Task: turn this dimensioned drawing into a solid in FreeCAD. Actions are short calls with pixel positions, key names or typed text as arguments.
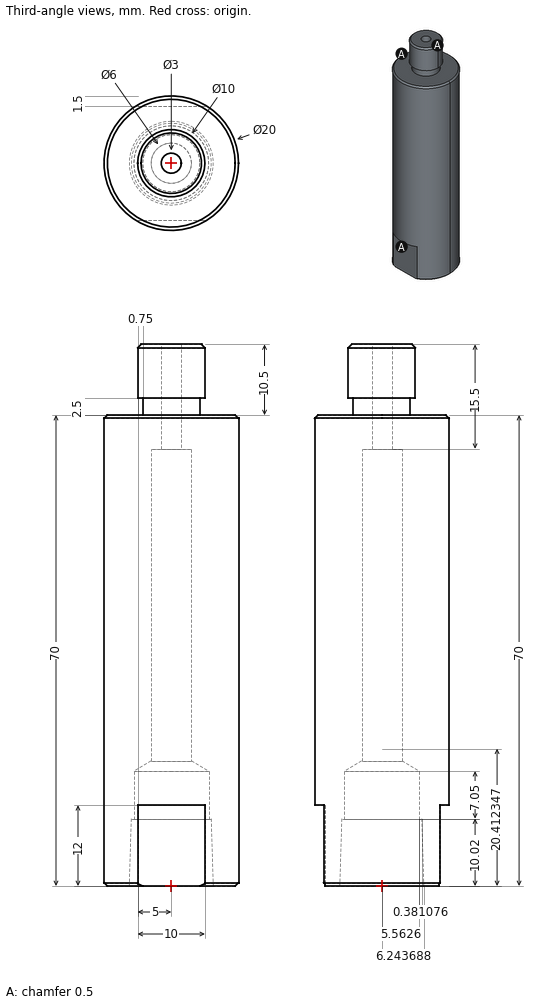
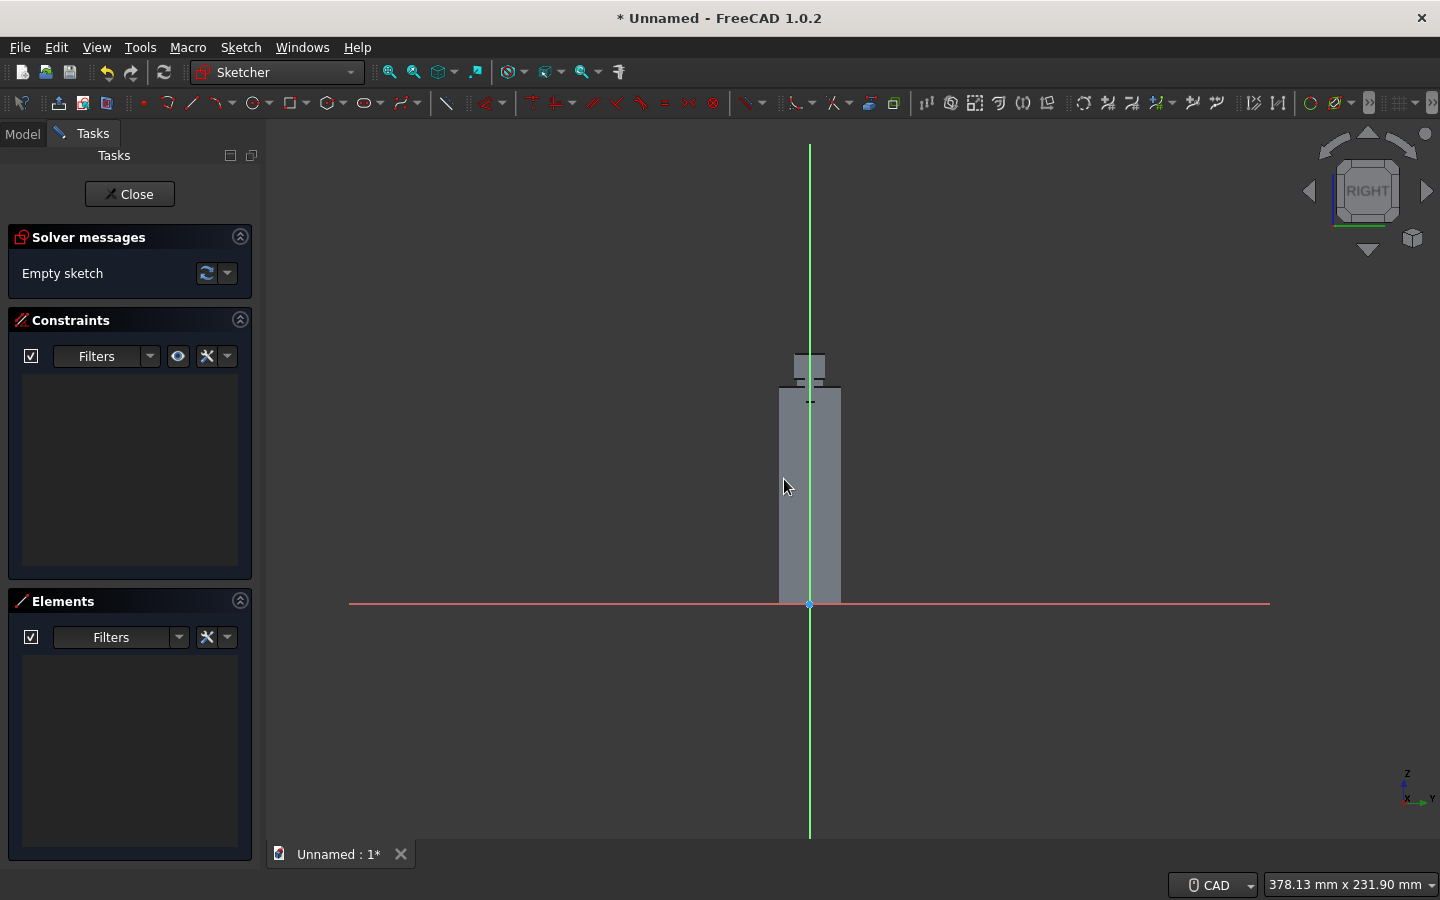
scroll(825, 587, up, 10)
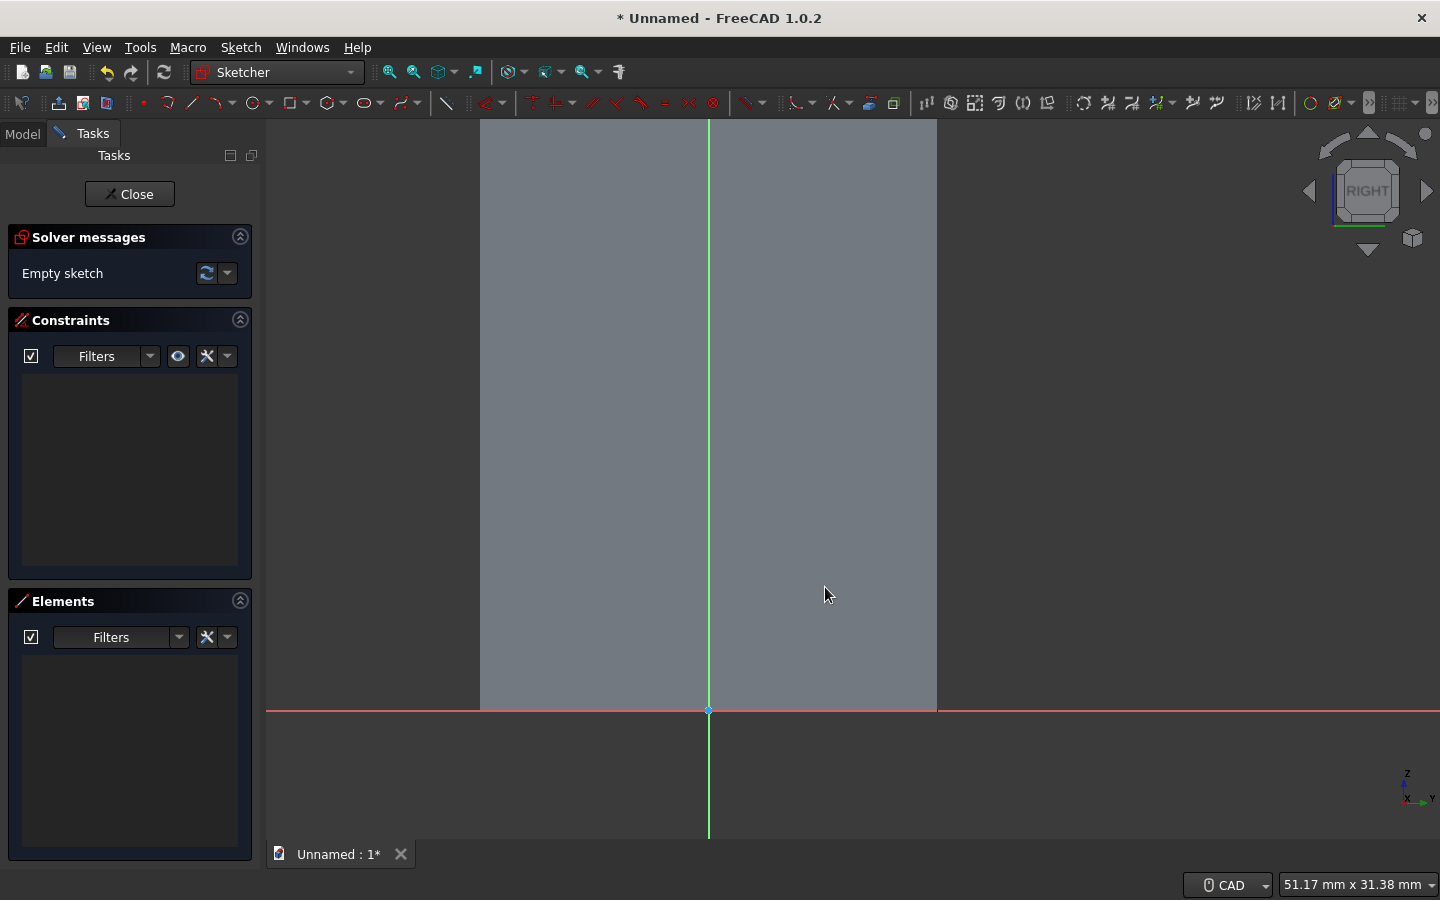
key(g)
key(m)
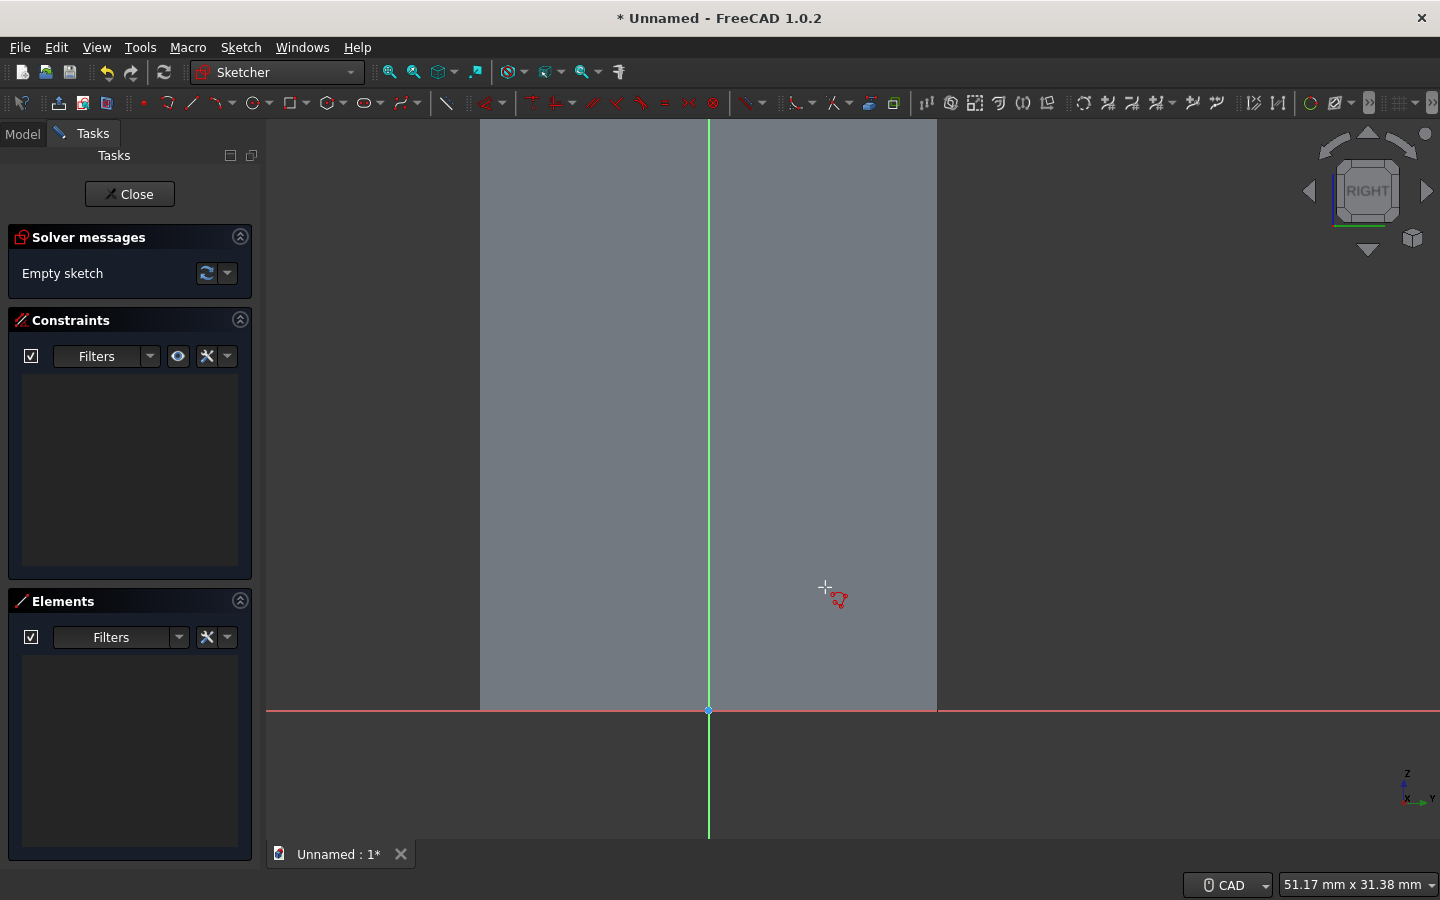
click(709, 711)
click(852, 702)
click(840, 481)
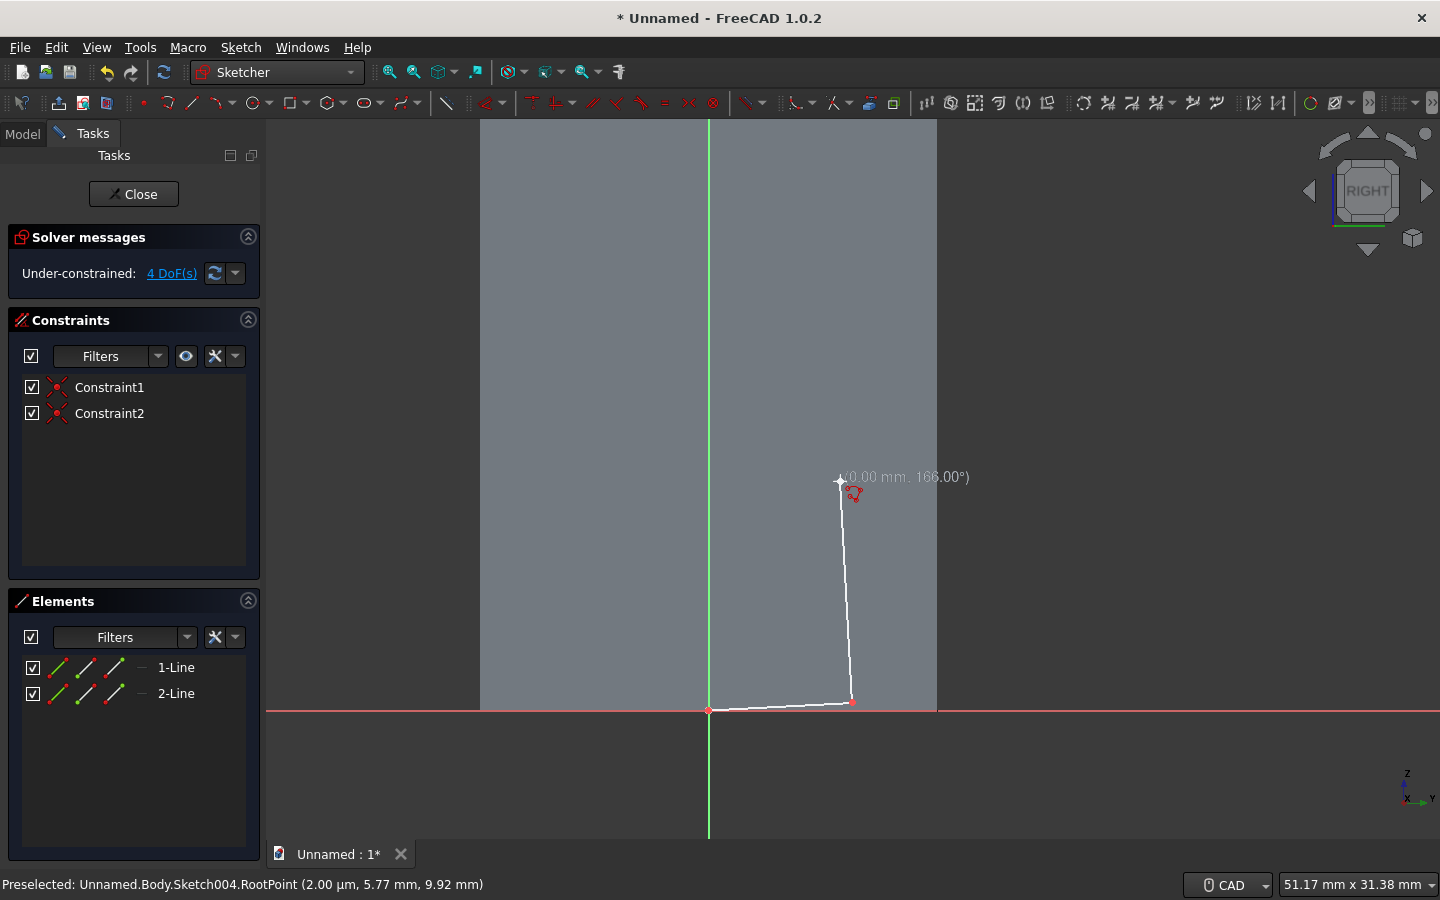
scroll(836, 481, up, 3)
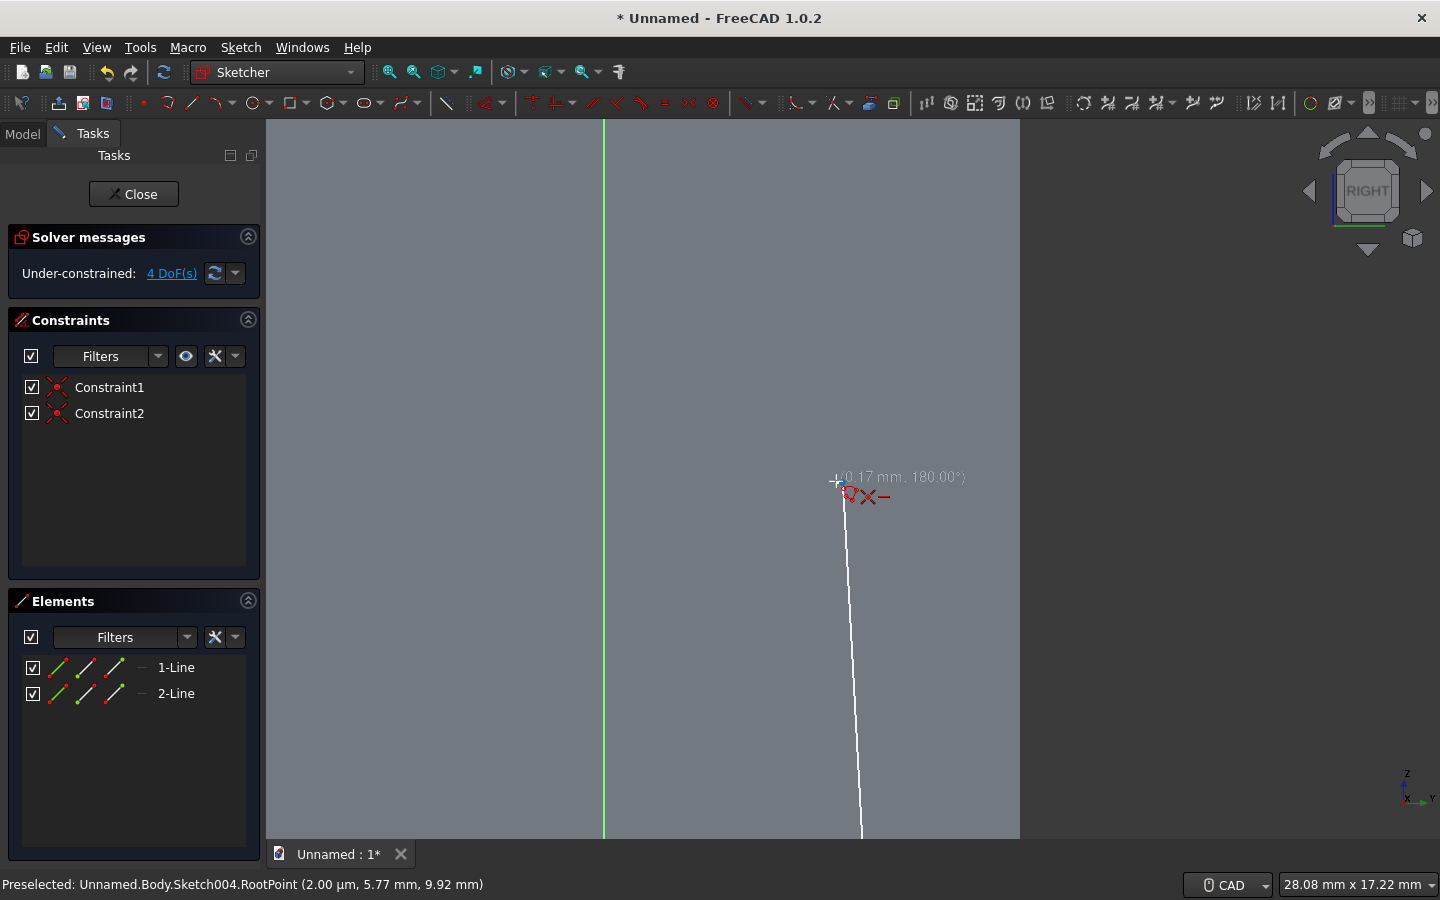
click(836, 481)
click(836, 185)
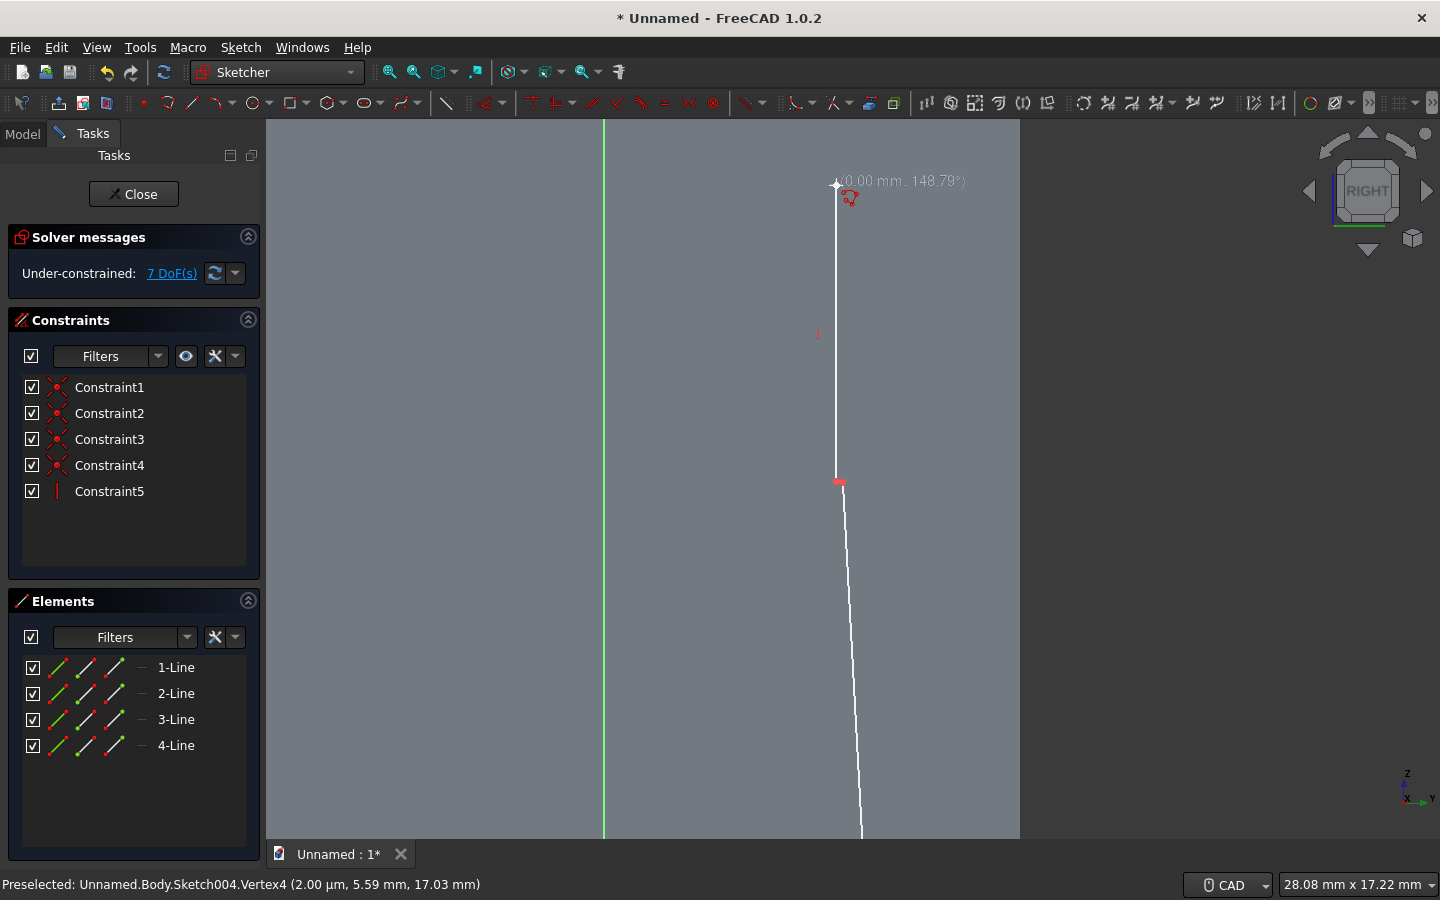
scroll(846, 487, down, 3)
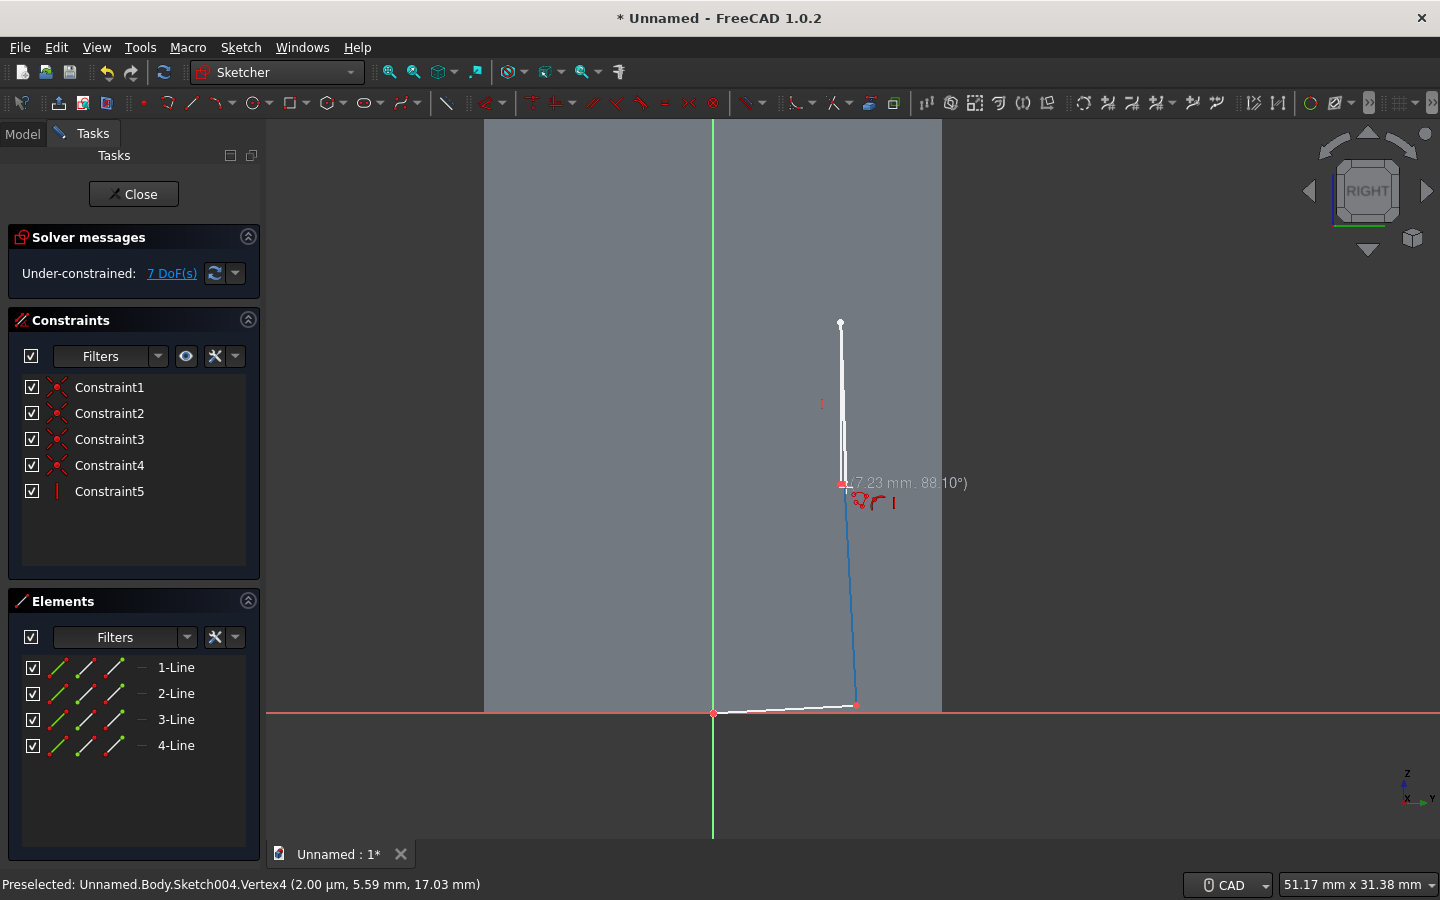
click(722, 245)
click(713, 713)
key(Escape)
key(Escape)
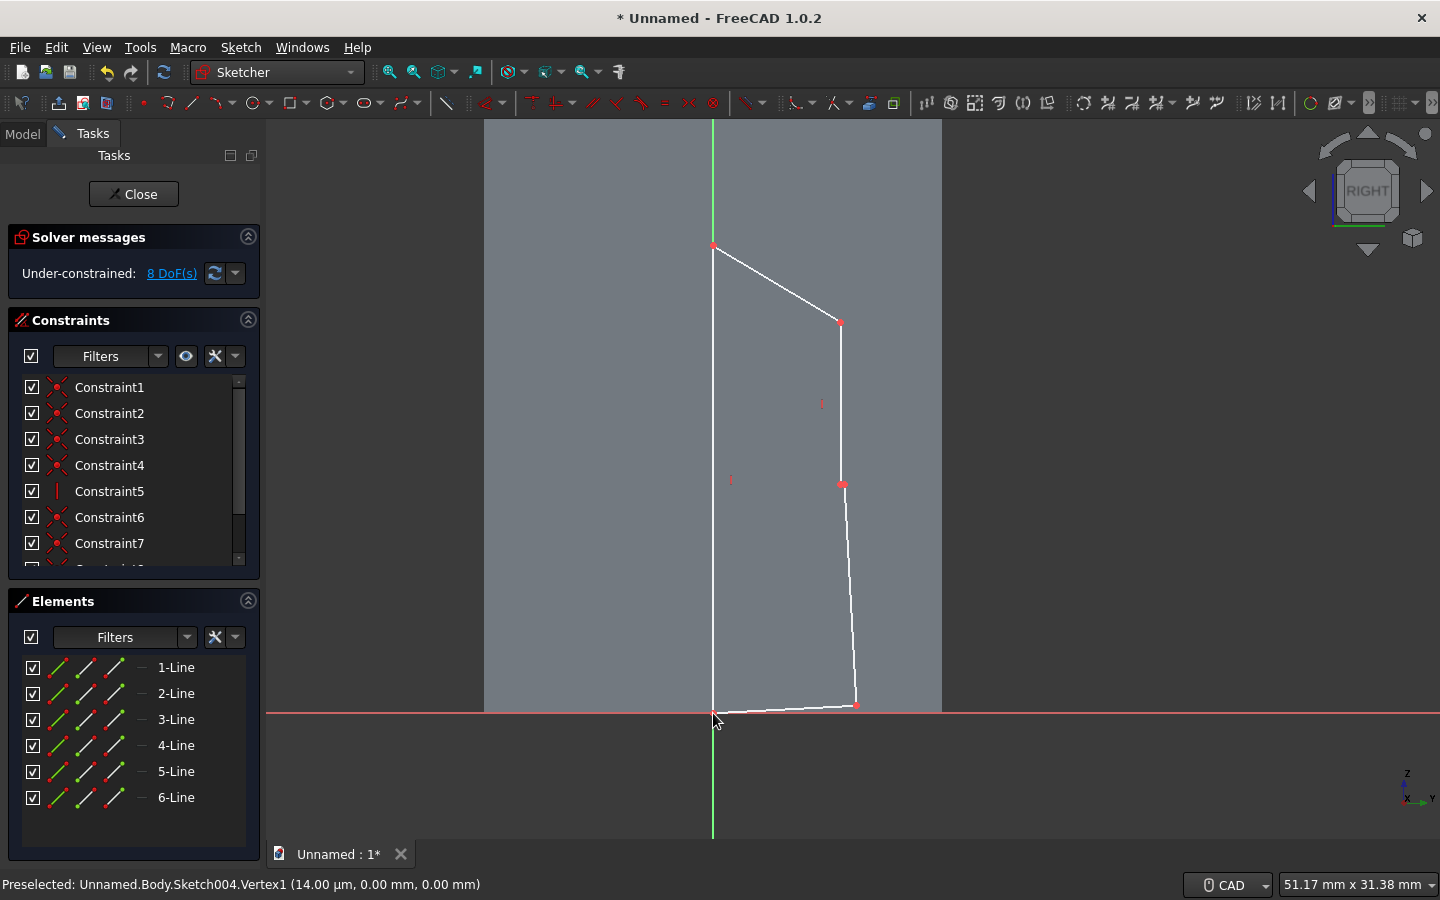
click(756, 711)